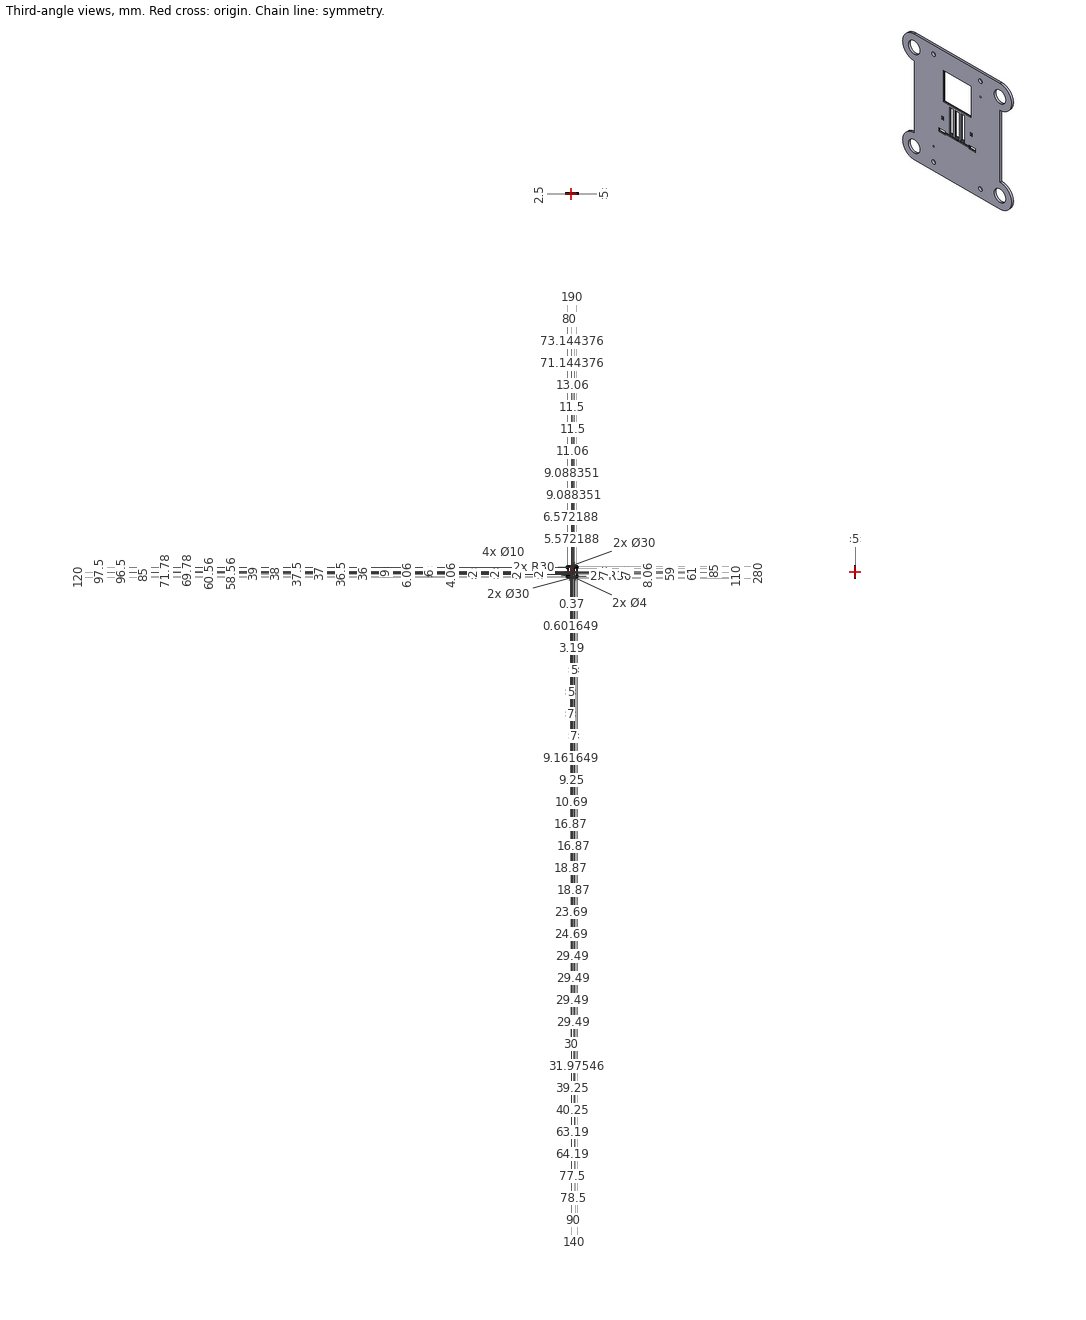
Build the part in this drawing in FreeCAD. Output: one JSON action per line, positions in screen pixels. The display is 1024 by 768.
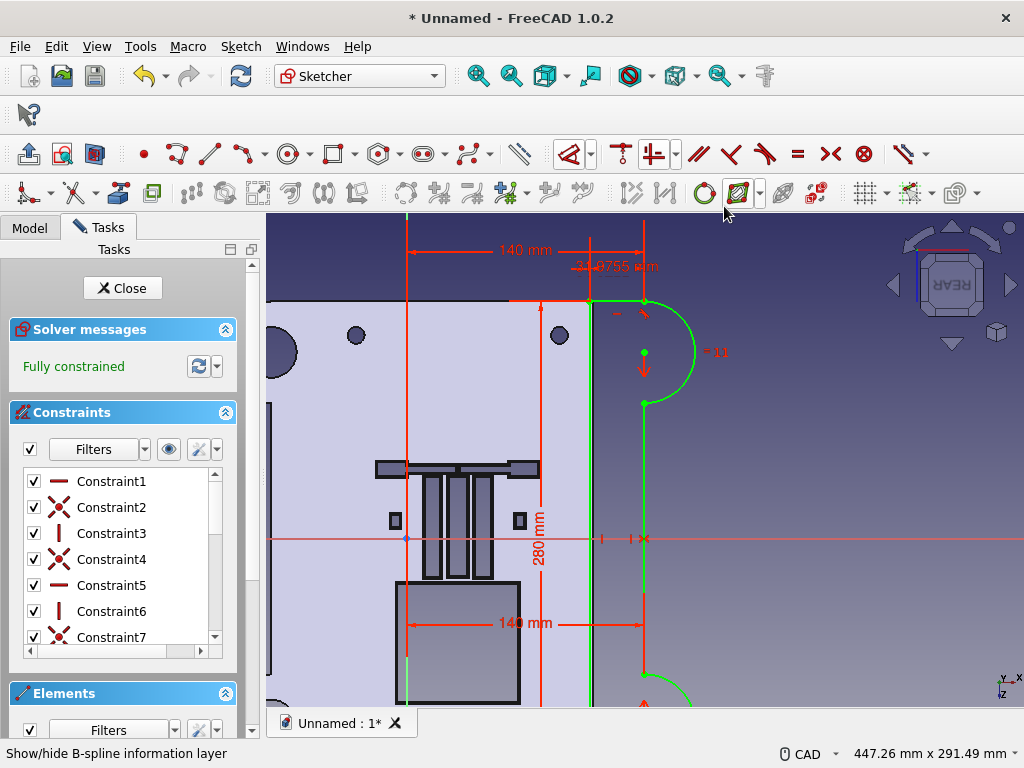
{"action": "left_click", "coordinate": [123, 288]}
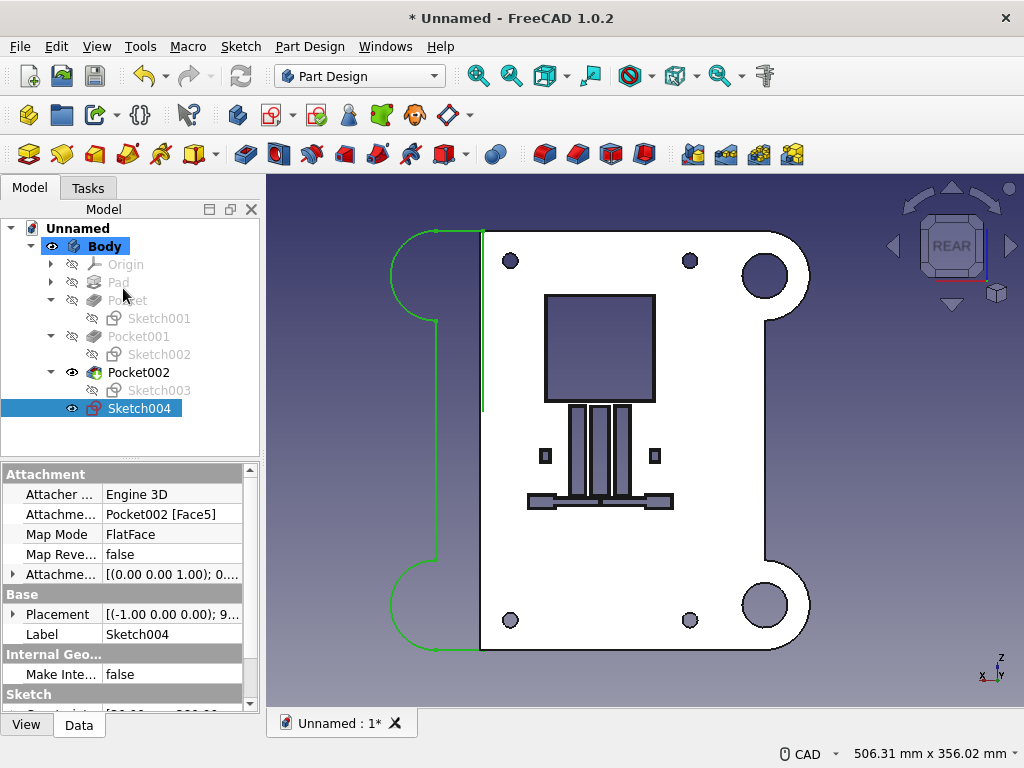
{"action": "left_click", "coordinate": [29, 154]}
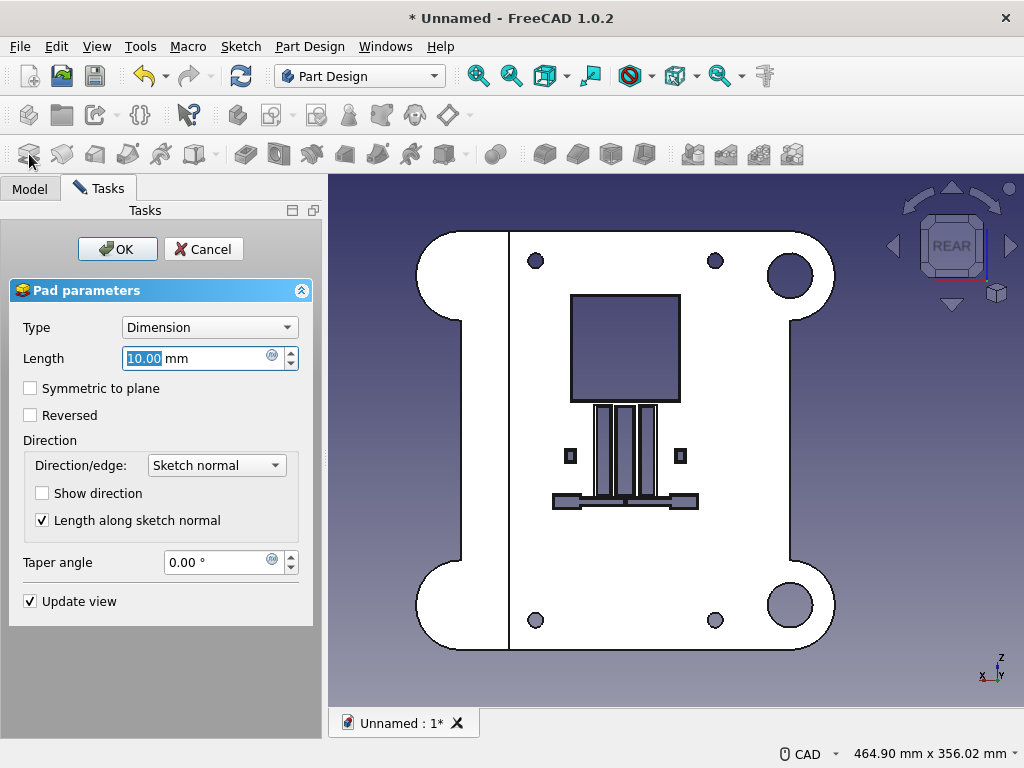
{"action": "type", "text": "5"}
{"action": "key", "text": "Tab"}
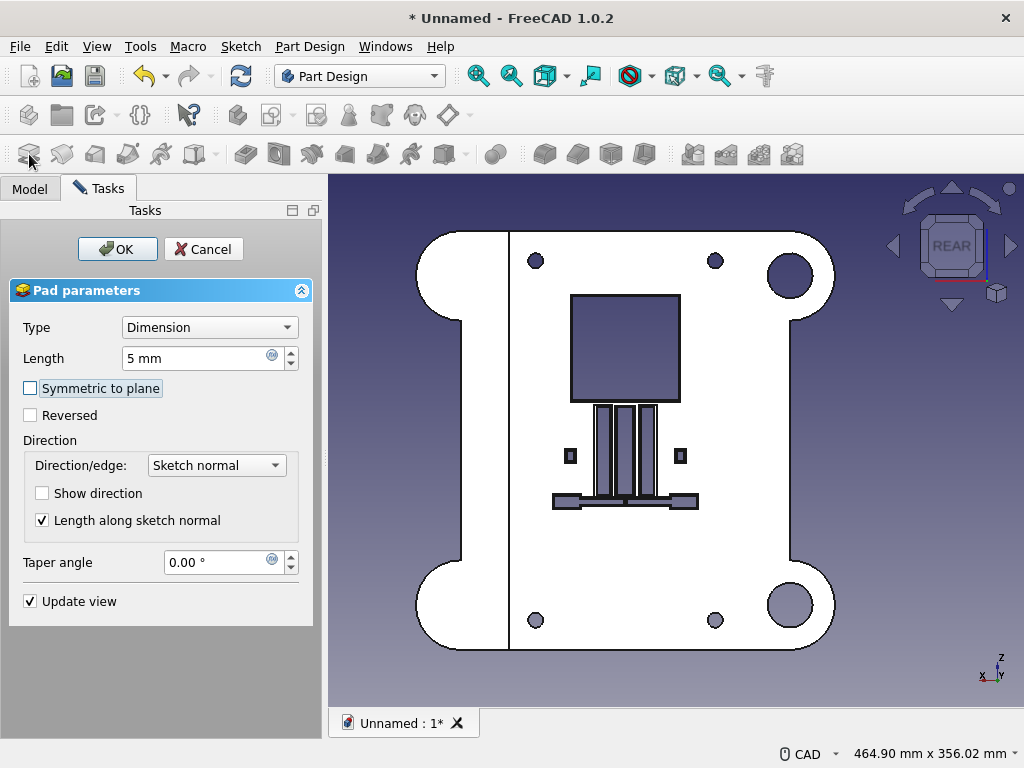
{"action": "left_click", "coordinate": [31, 415]}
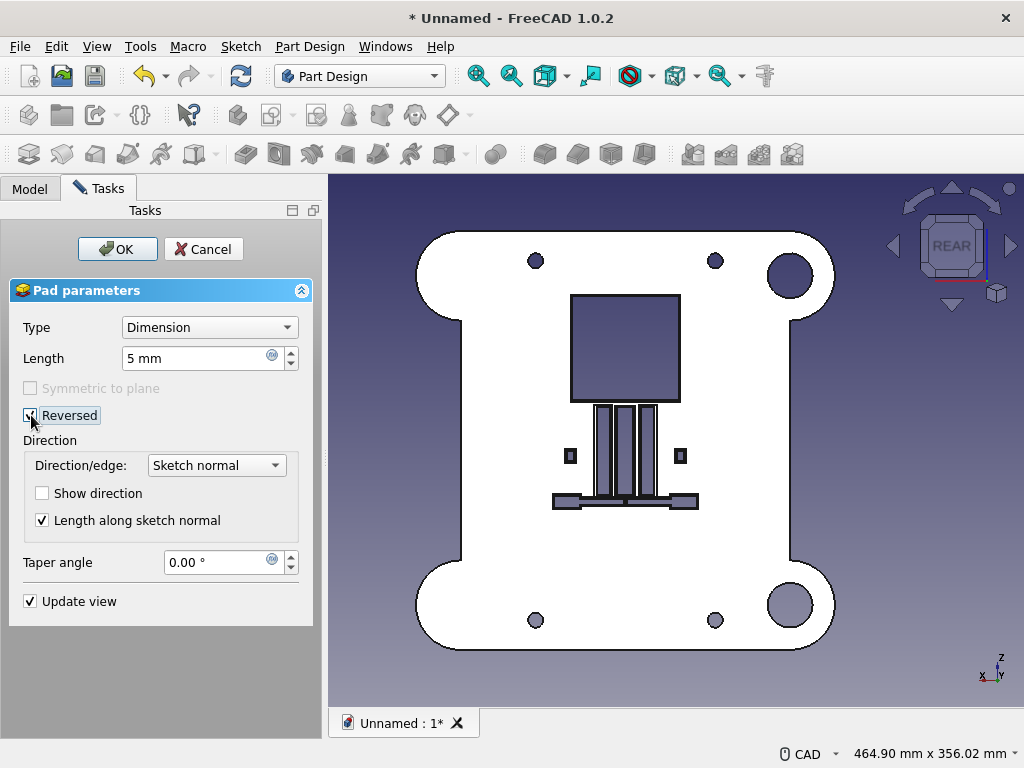
{"action": "left_click", "coordinate": [118, 249]}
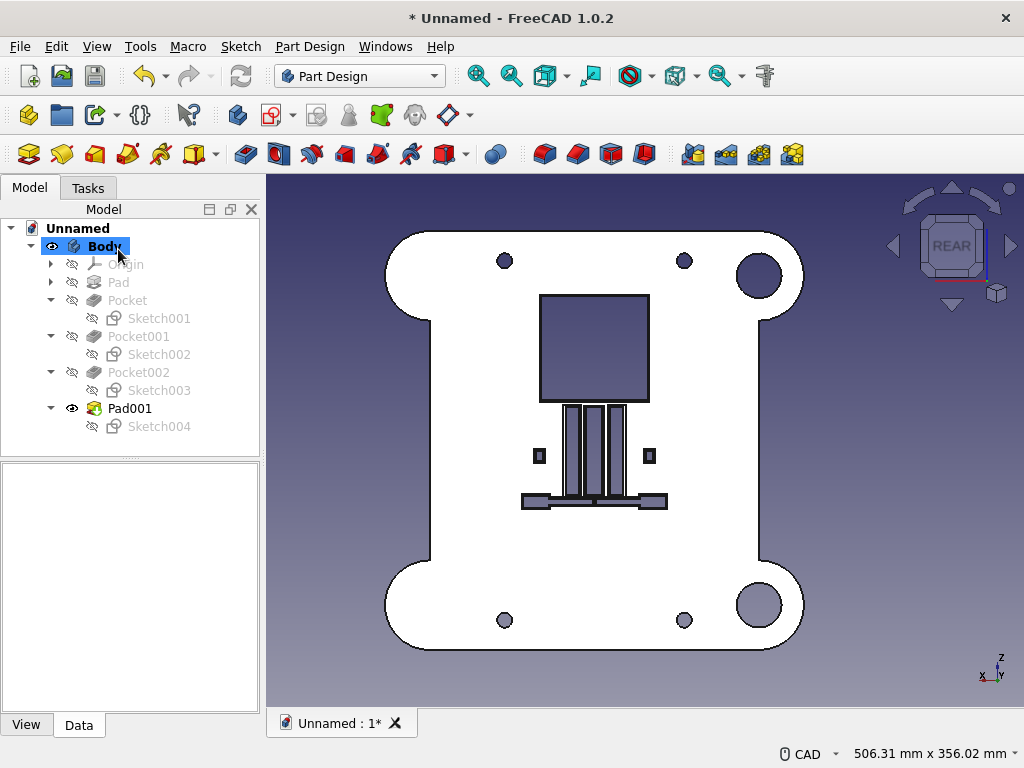
{"action": "left_click", "coordinate": [594, 559]}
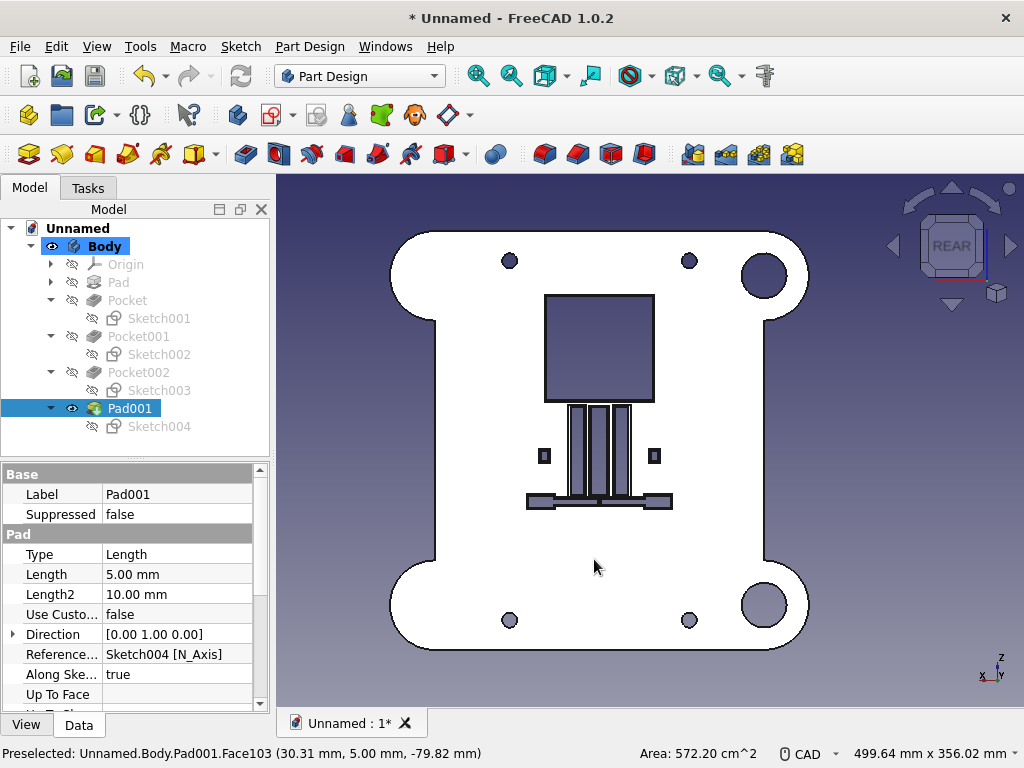
{"action": "left_click", "coordinate": [270, 116]}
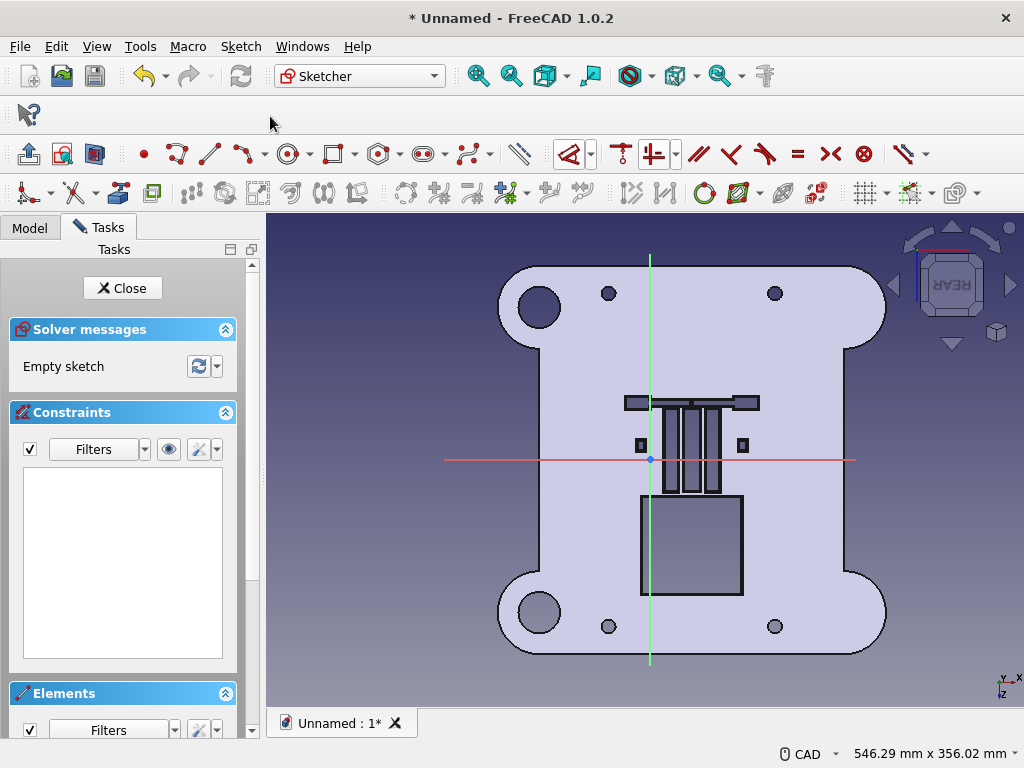
{"action": "scroll", "coordinate": [294, 460], "scroll_direction": "down", "scroll_amount": 1}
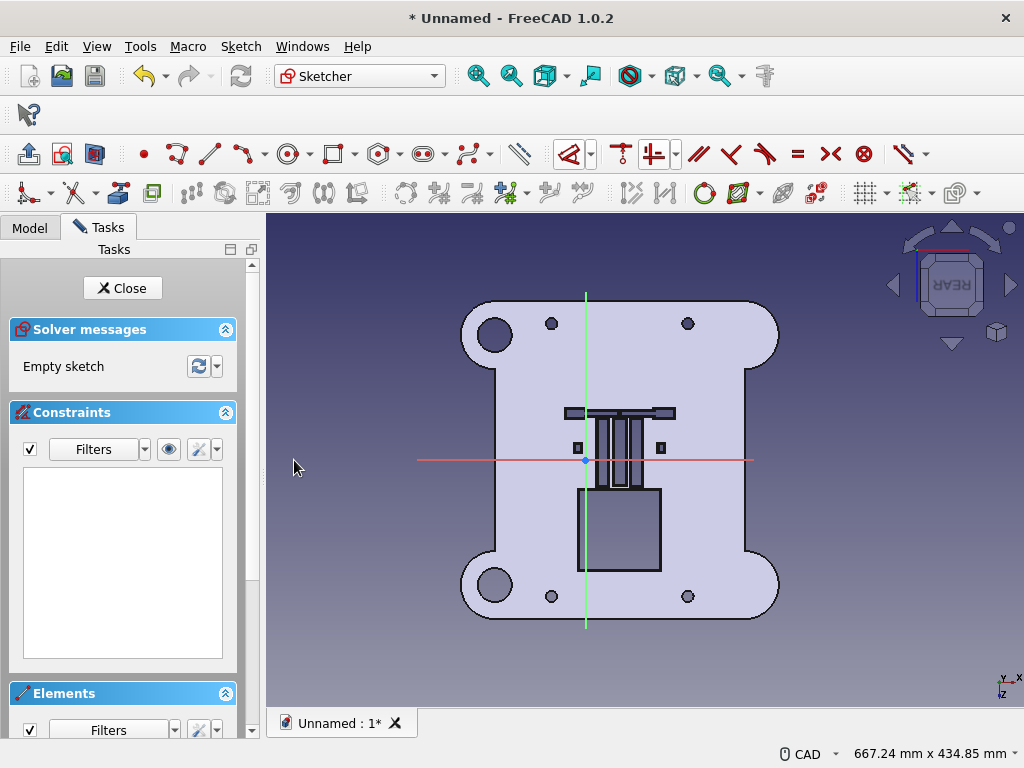
{"action": "key", "text": "g c"}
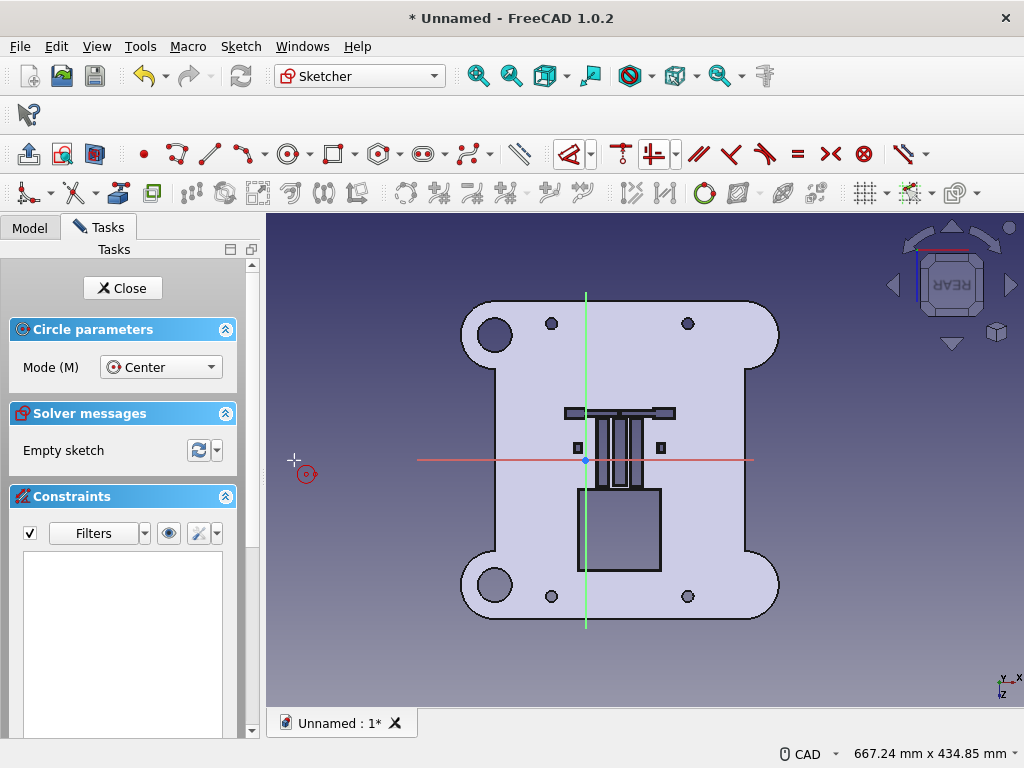
{"action": "scroll", "coordinate": [745, 335], "scroll_direction": "up", "scroll_amount": 2}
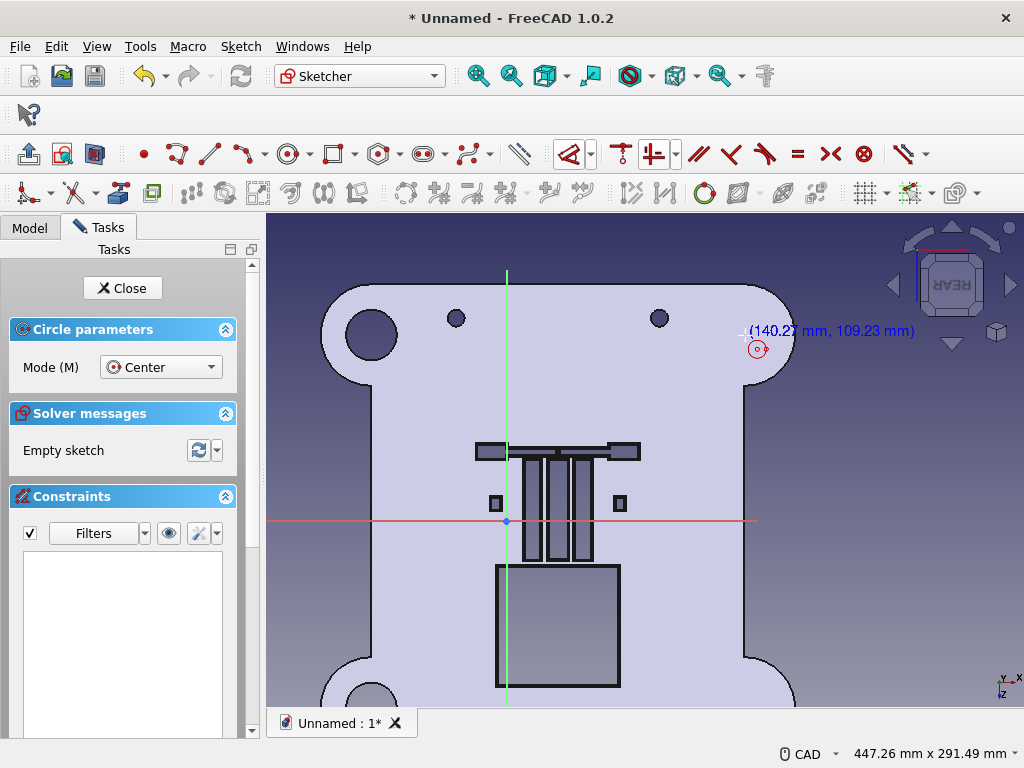
{"action": "left_click", "coordinate": [744, 335]}
{"action": "left_click", "coordinate": [762, 317]}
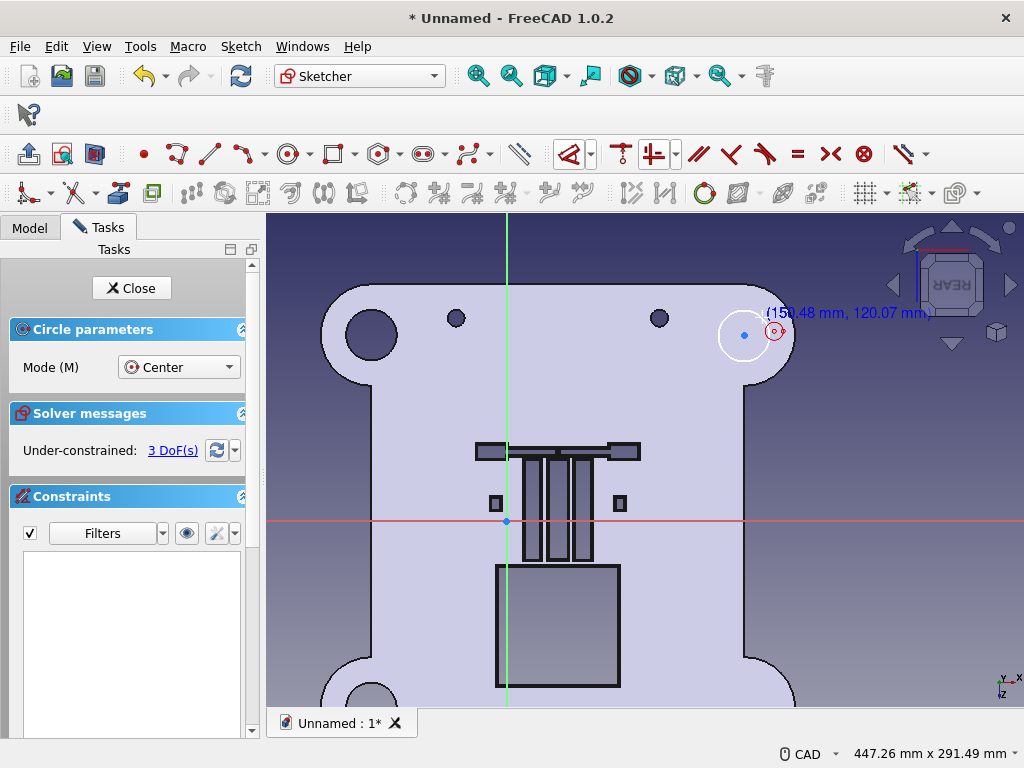
{"action": "scroll", "coordinate": [451, 335], "scroll_direction": "down", "scroll_amount": 2}